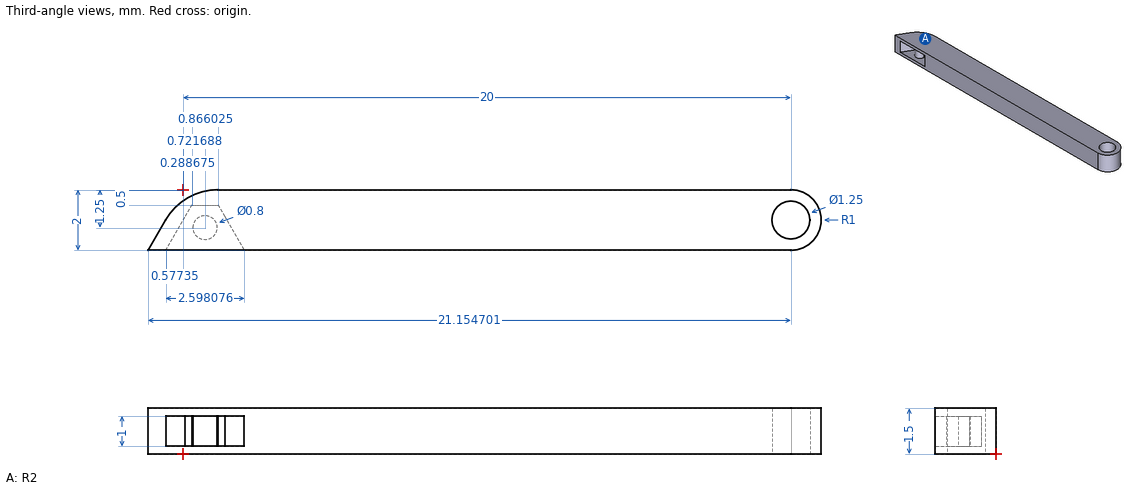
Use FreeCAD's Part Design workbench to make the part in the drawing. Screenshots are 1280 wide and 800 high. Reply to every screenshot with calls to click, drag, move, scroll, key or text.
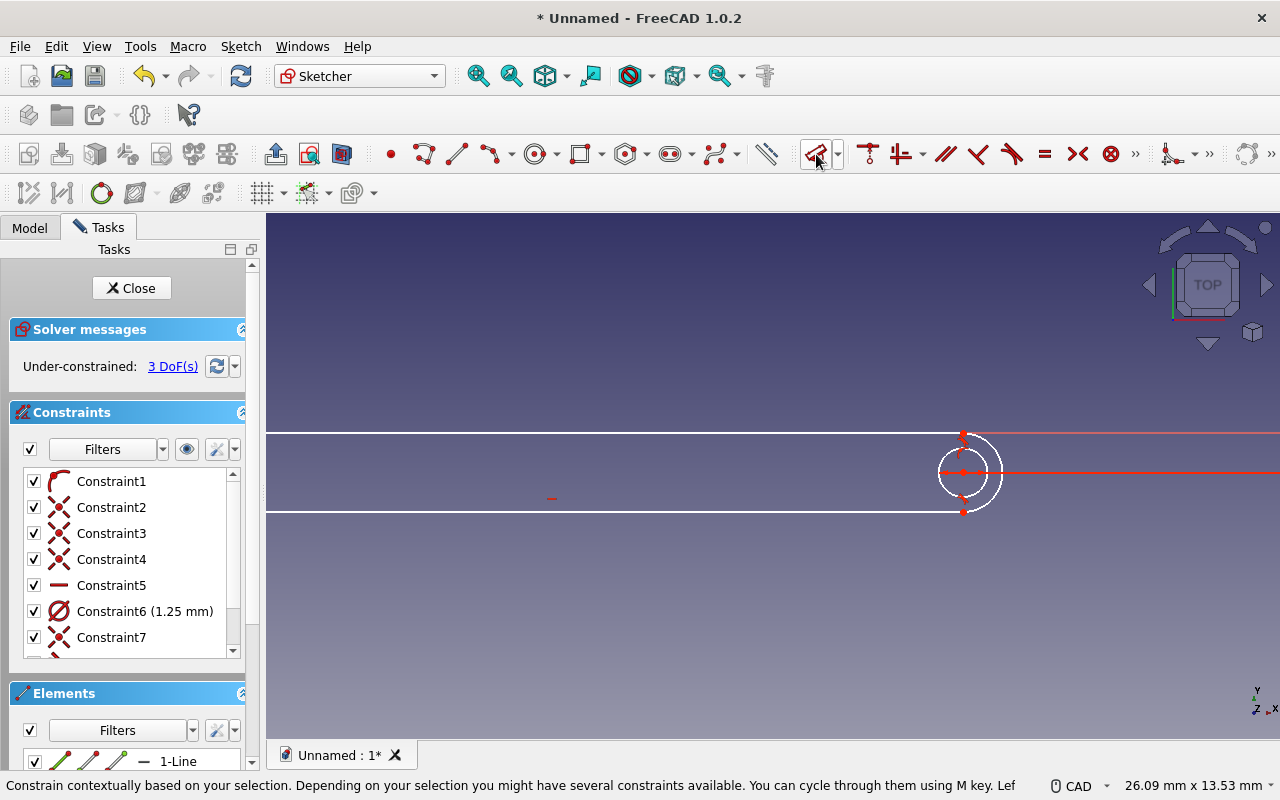
click(995, 496)
click(1021, 515)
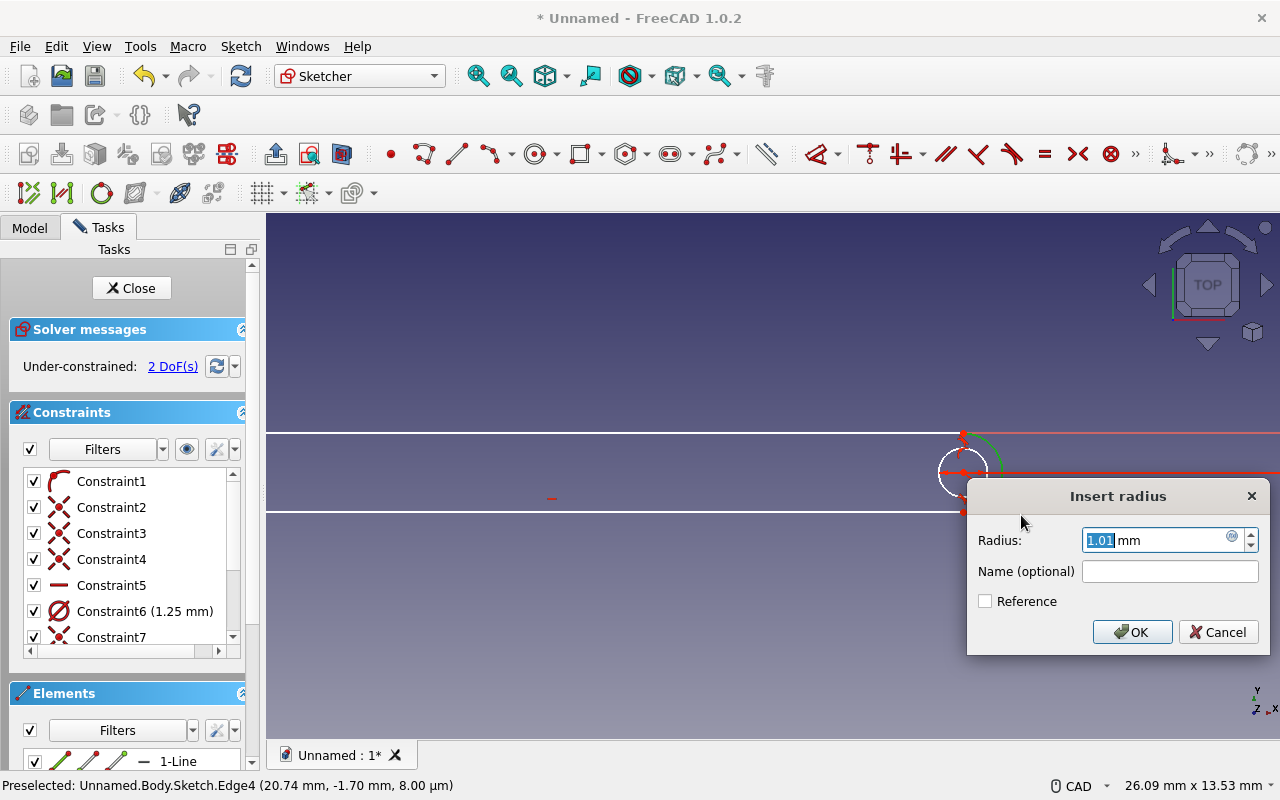
text(1)
key(Return)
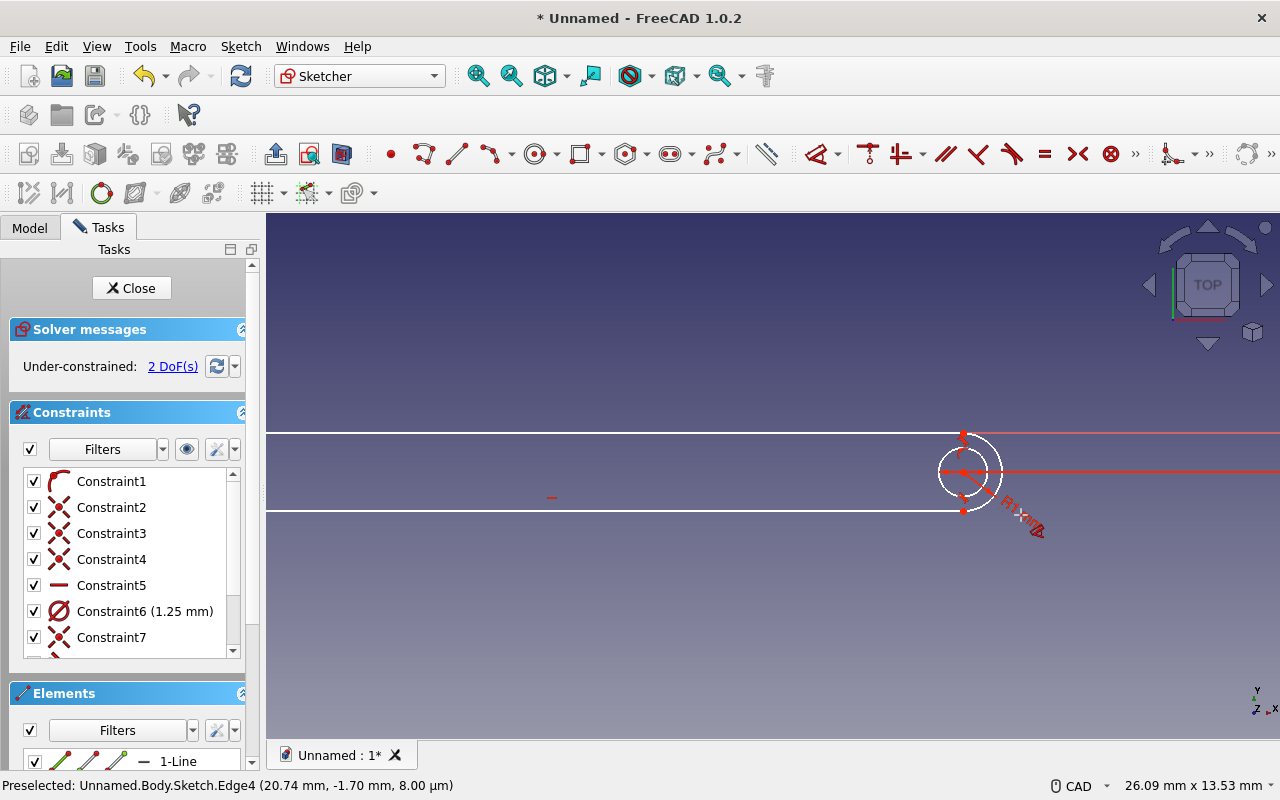
click(730, 433)
click(629, 399)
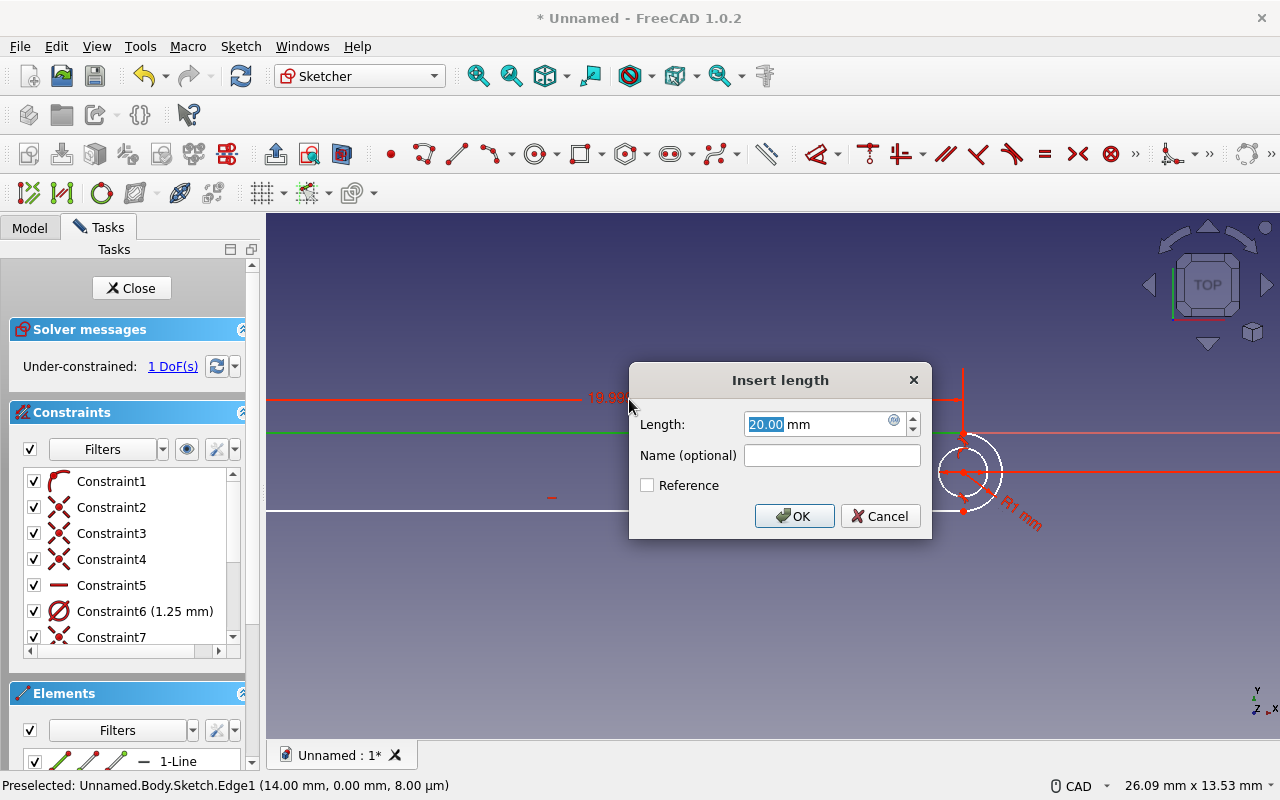
text(20)
key(Return)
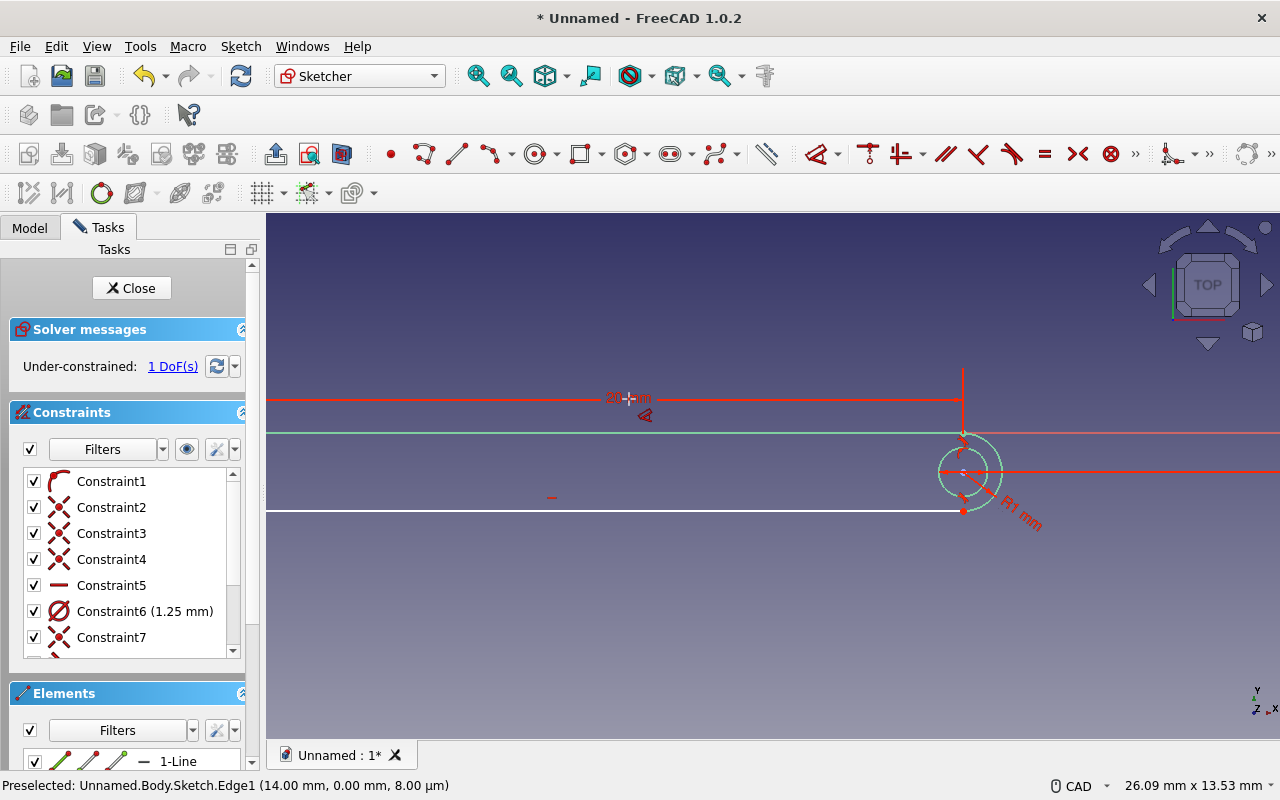
click(388, 511)
click(629, 545)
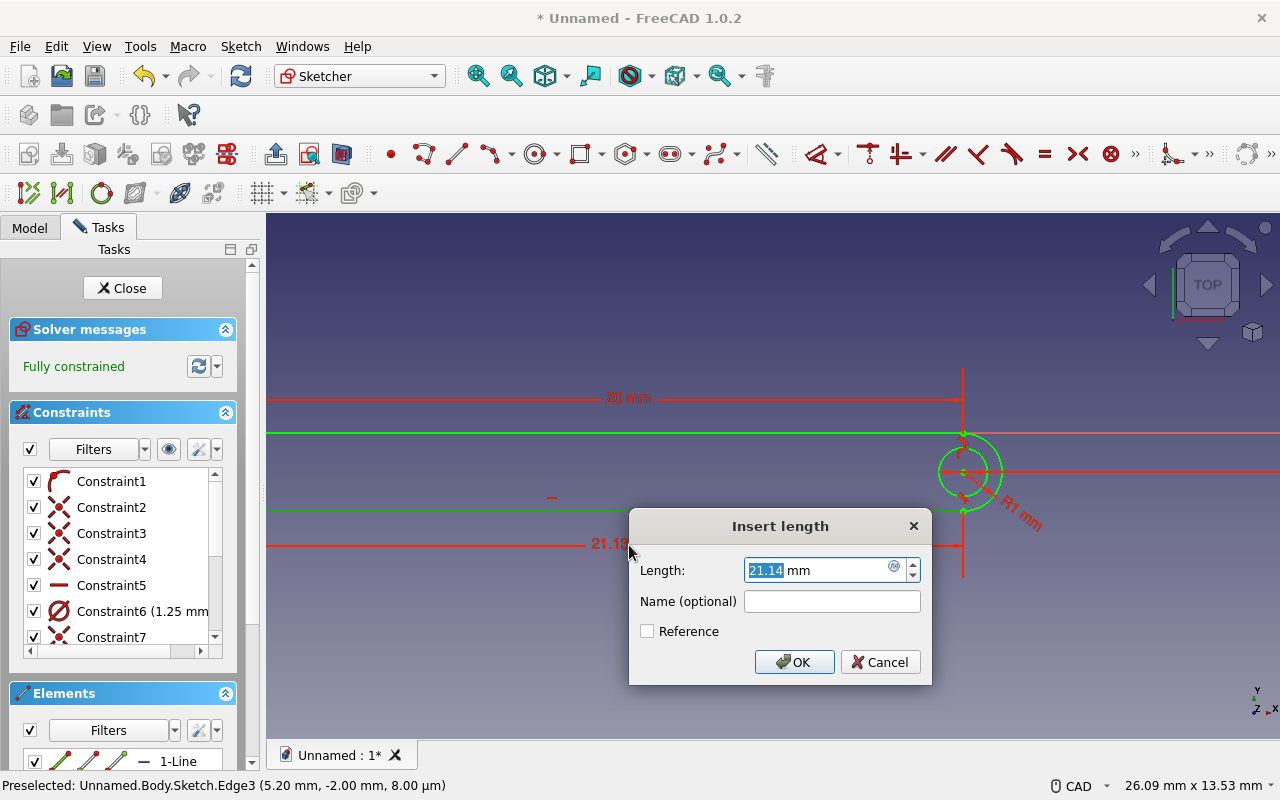
text(21.154701)
key(Return)
key(Escape)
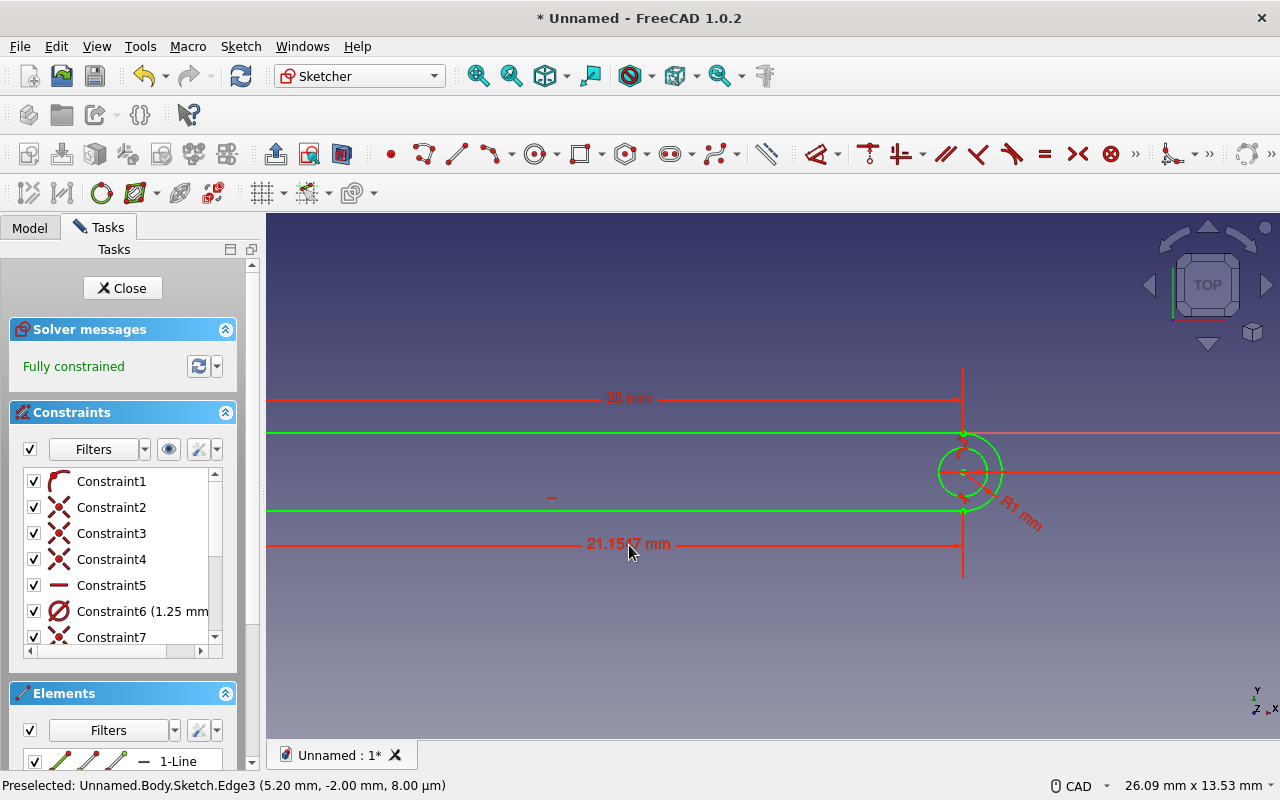
click(123, 288)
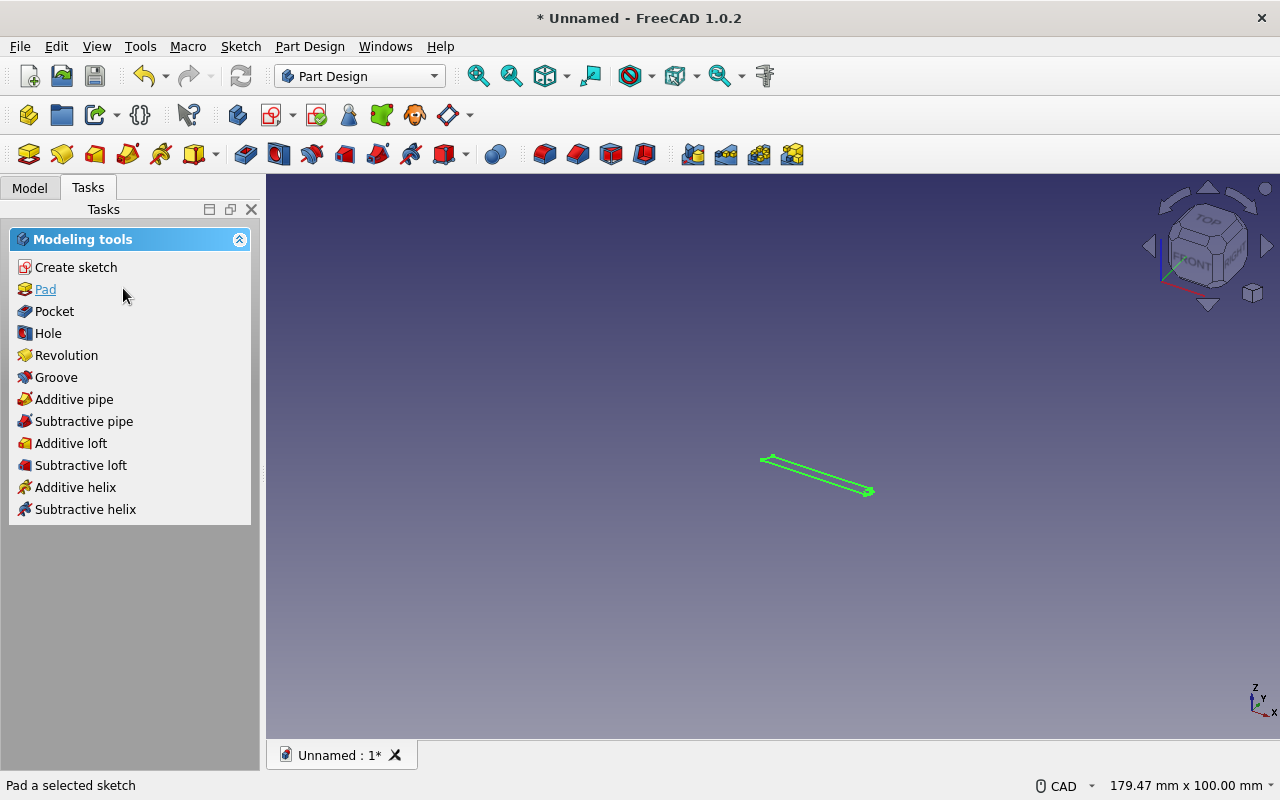
click(29, 154)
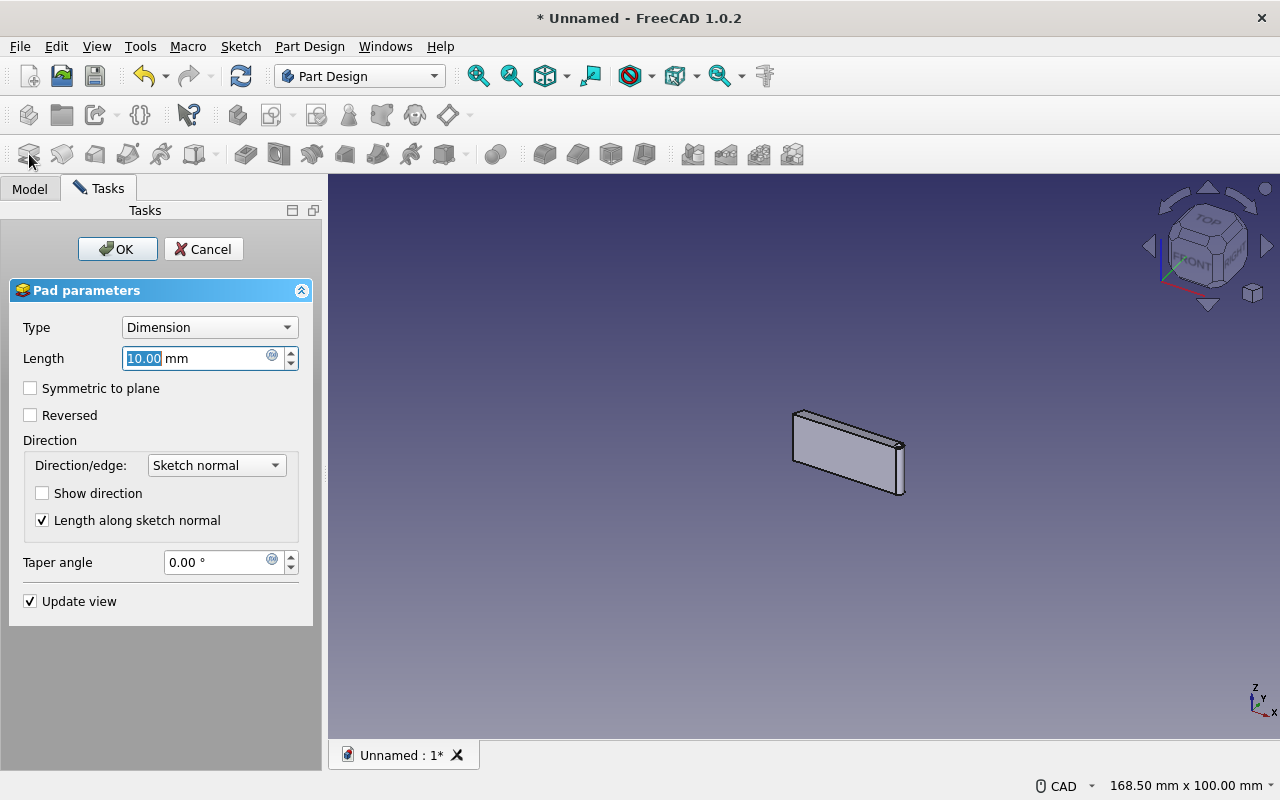
text(1.5)
key(Tab)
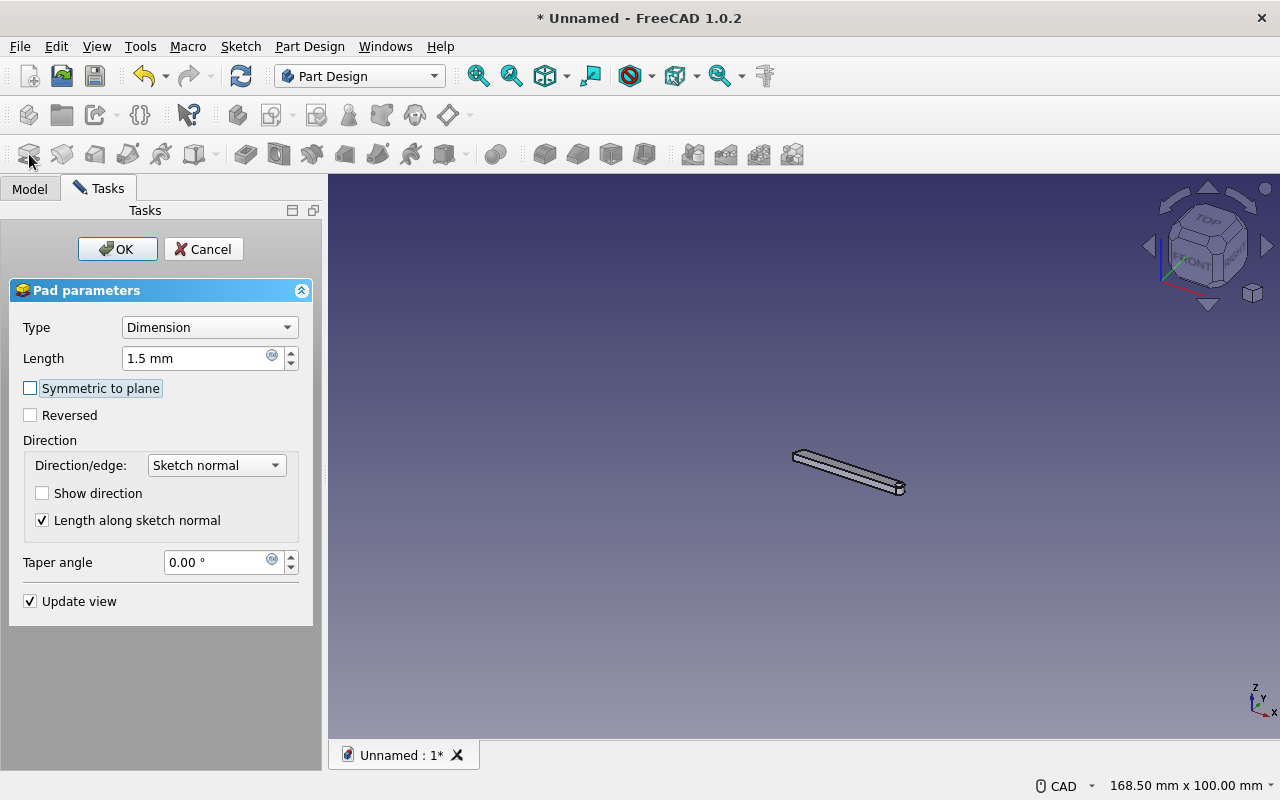
click(118, 249)